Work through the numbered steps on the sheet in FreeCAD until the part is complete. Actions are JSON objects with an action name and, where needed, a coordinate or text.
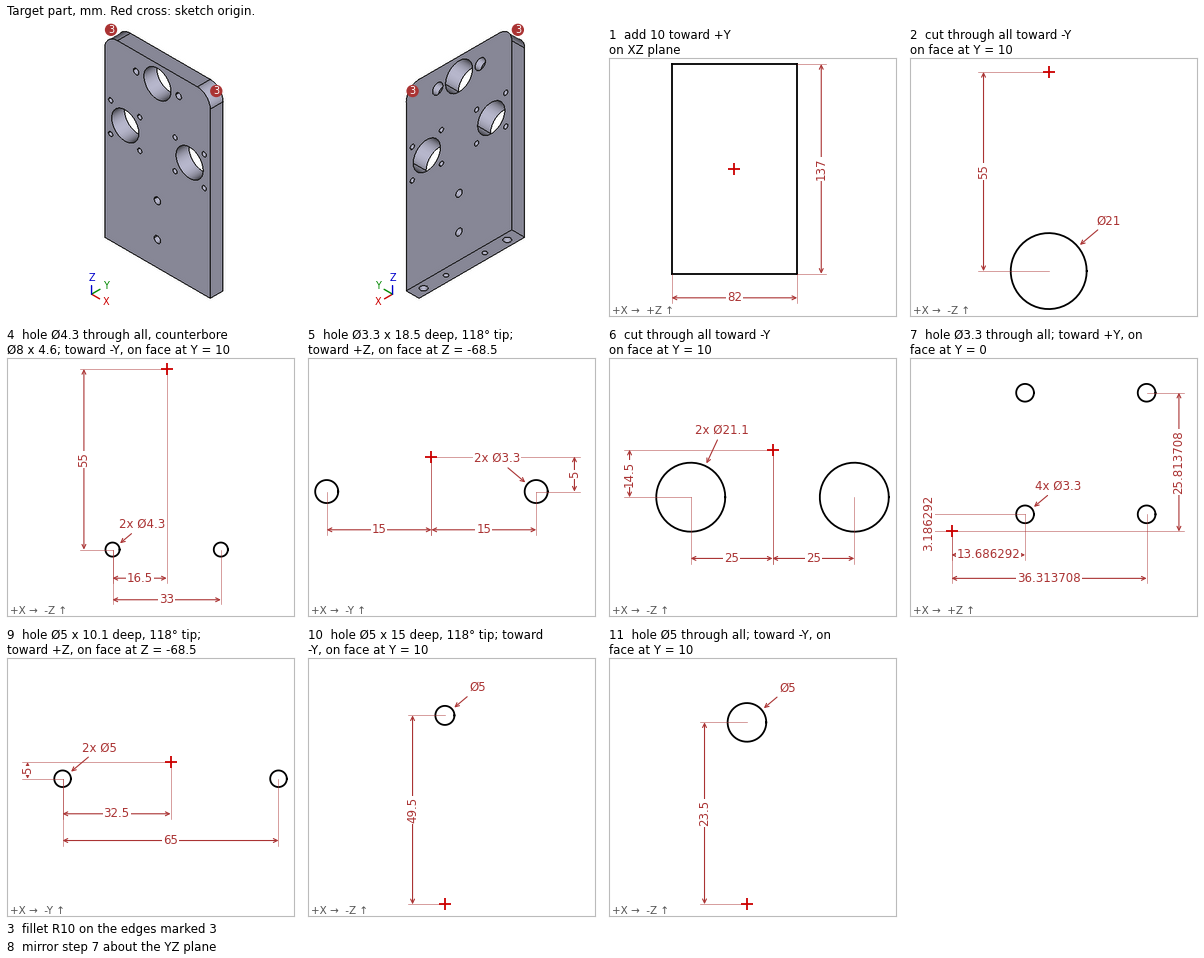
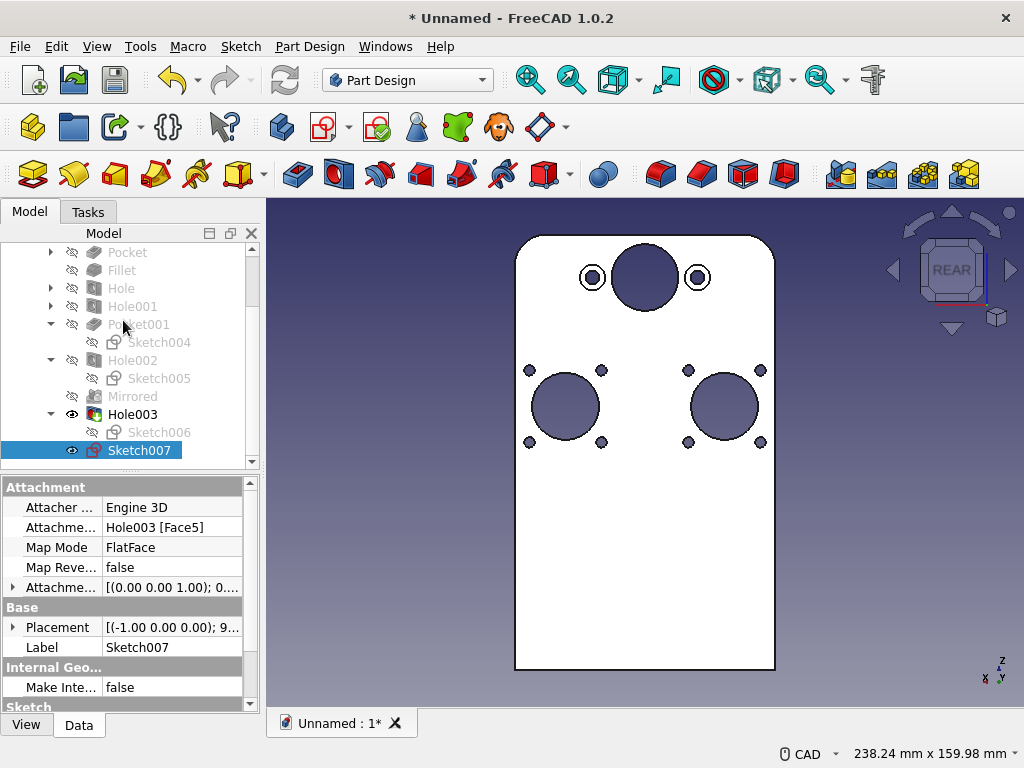
{"action": "left_click", "coordinate": [339, 174]}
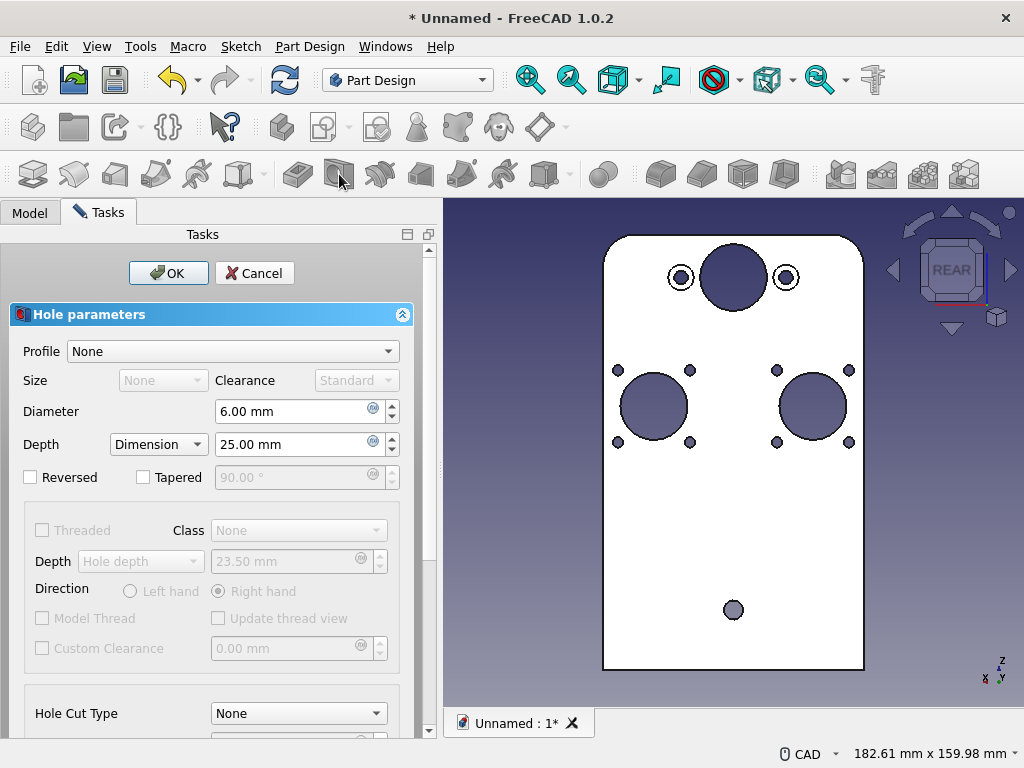
{"action": "triple_click", "coordinate": [300, 412]}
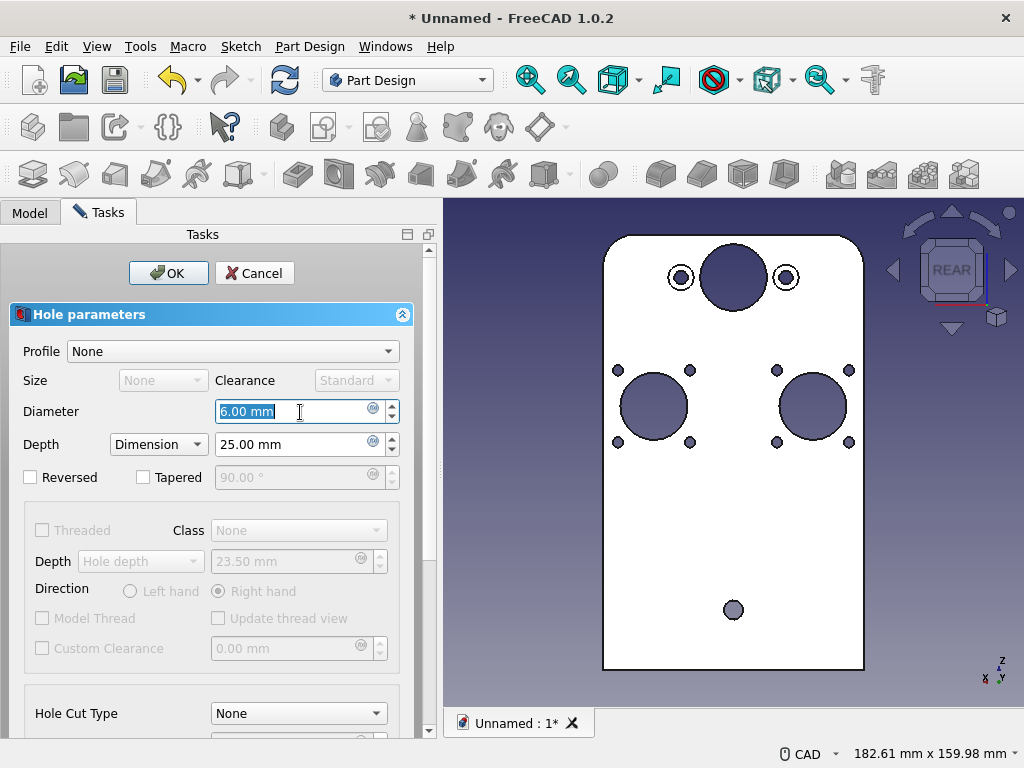
{"action": "type", "text": "5"}
{"action": "key", "text": "Tab"}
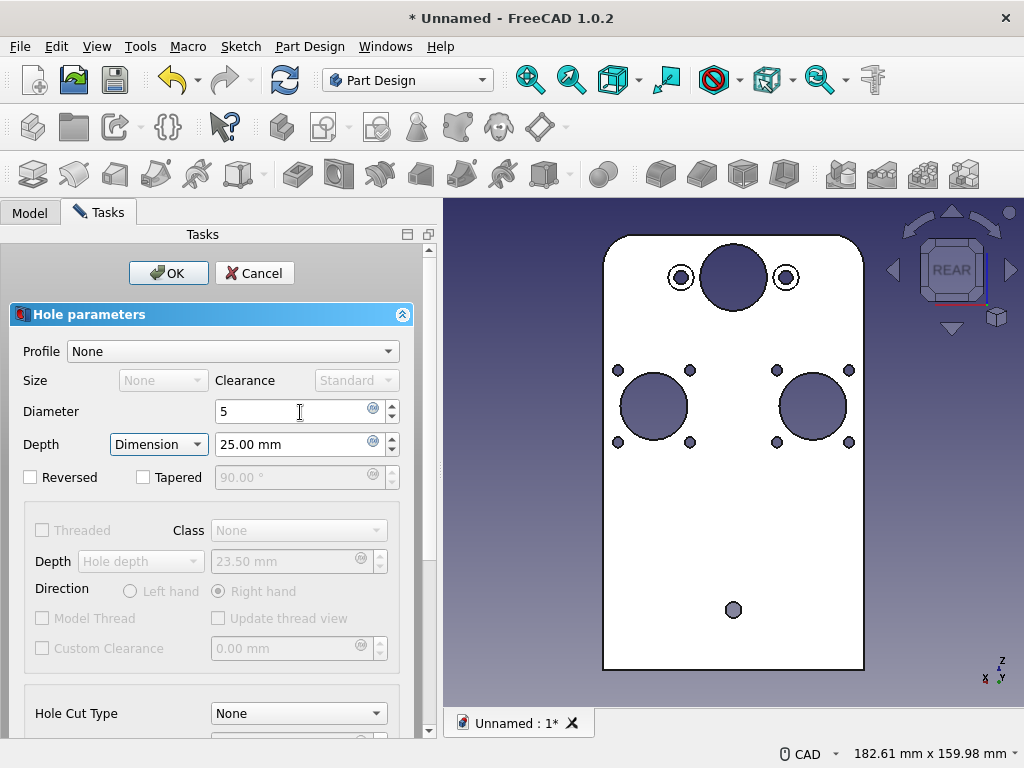
{"action": "triple_click", "coordinate": [300, 444]}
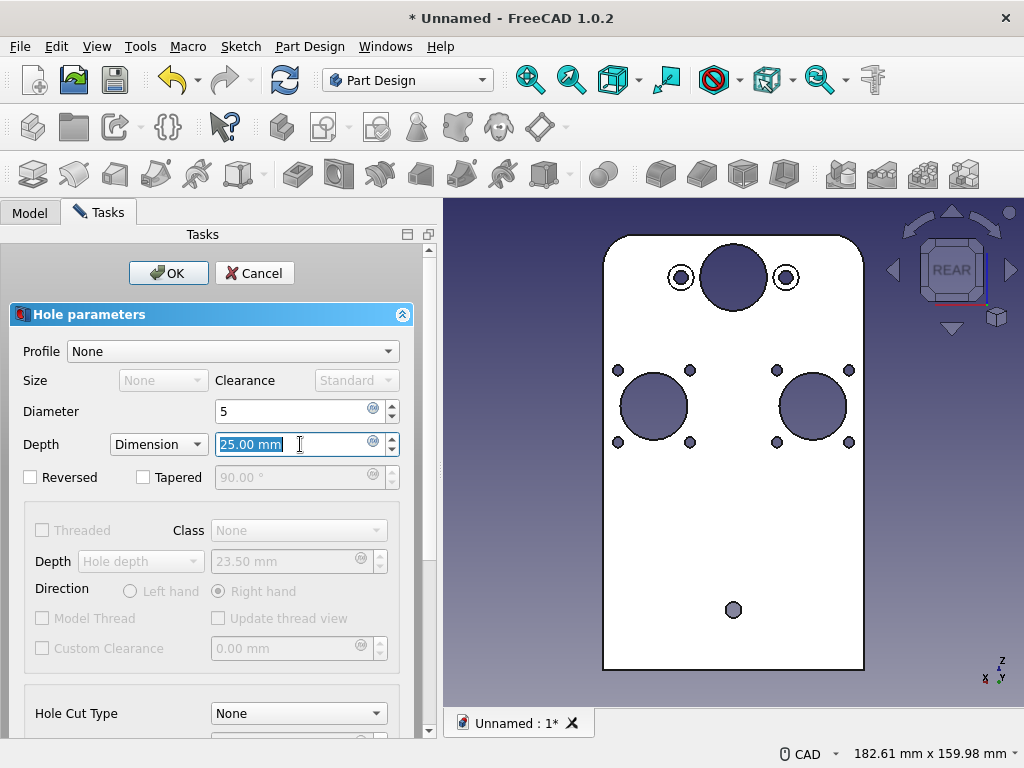
{"action": "type", "text": "15"}
{"action": "key", "text": "Tab"}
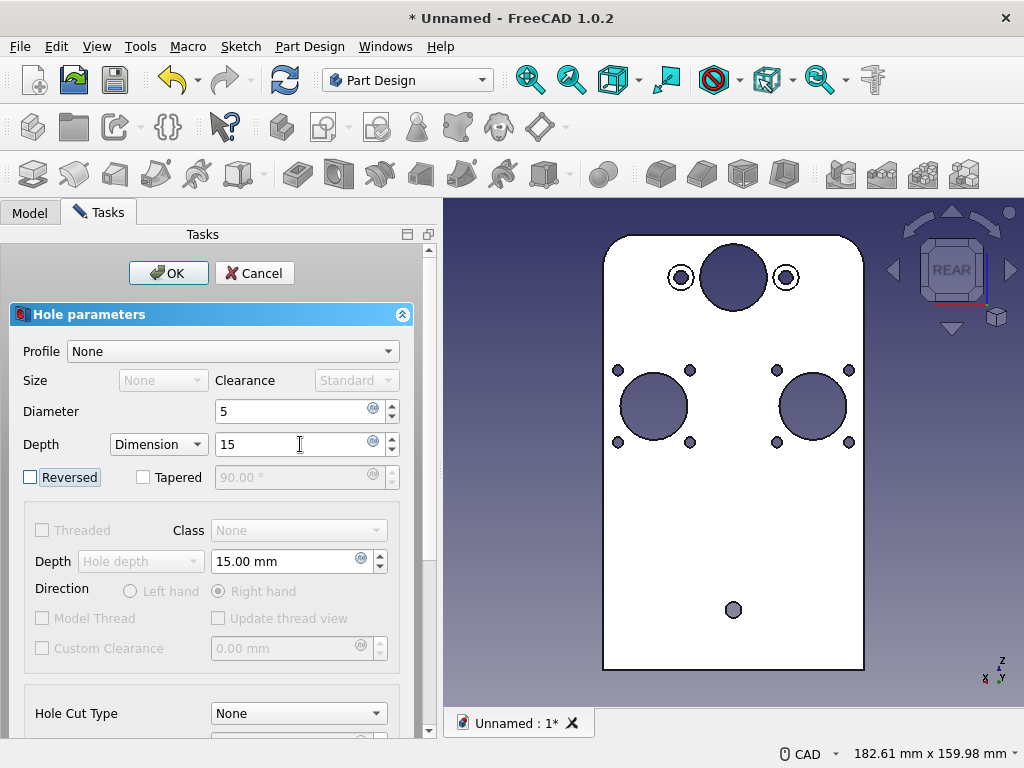
{"action": "left_click", "coordinate": [169, 273]}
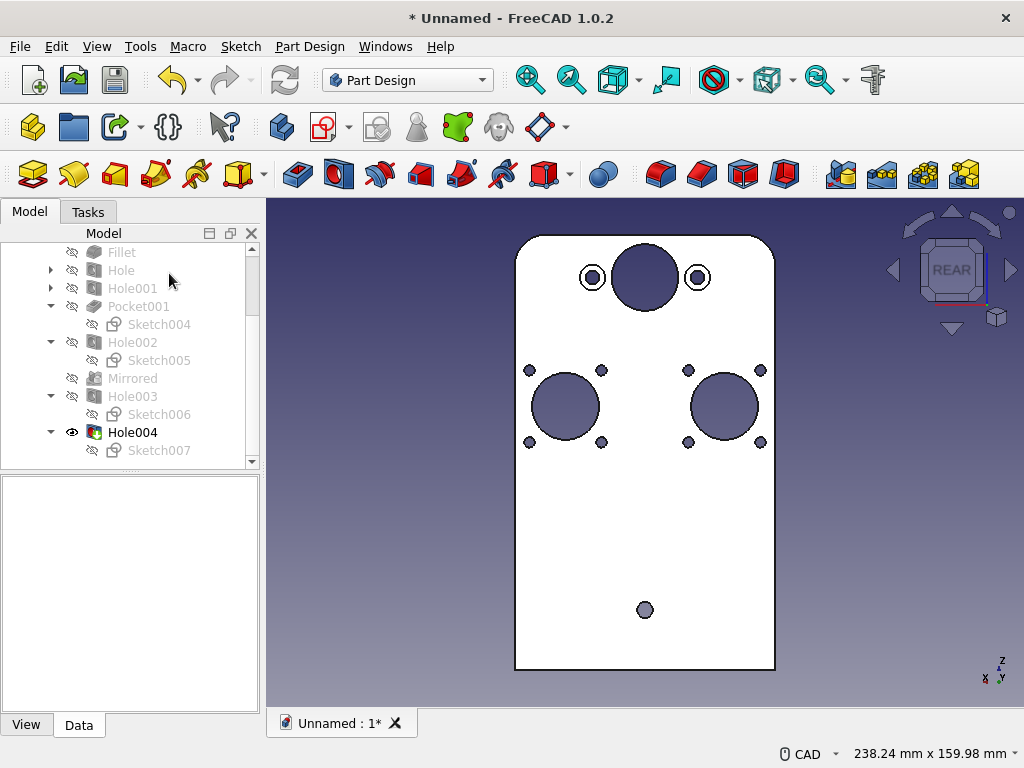
{"action": "left_click", "coordinate": [645, 514]}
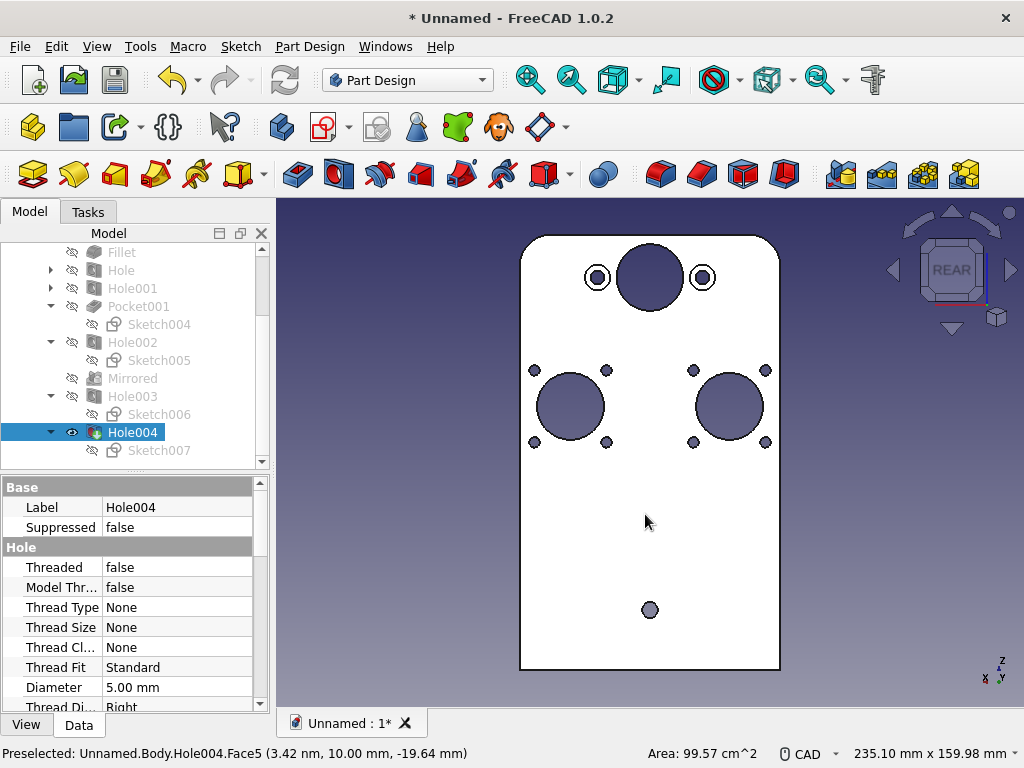
{"action": "left_click", "coordinate": [322, 128]}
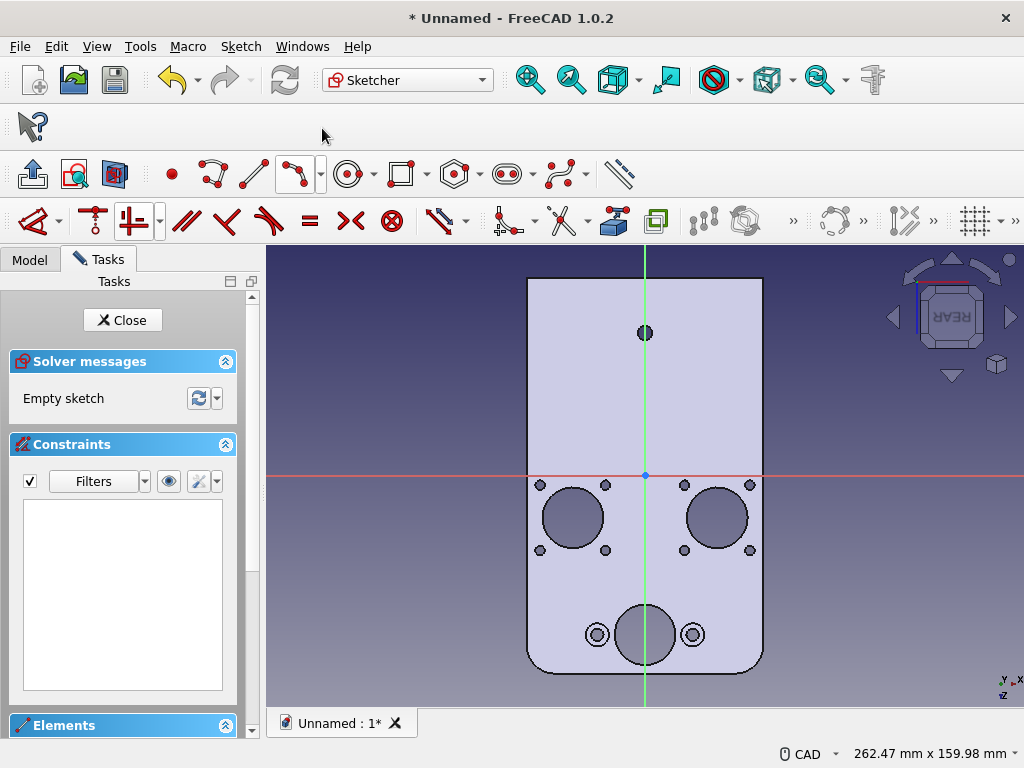
{"action": "scroll", "coordinate": [649, 405], "scroll_direction": "up", "scroll_amount": 15}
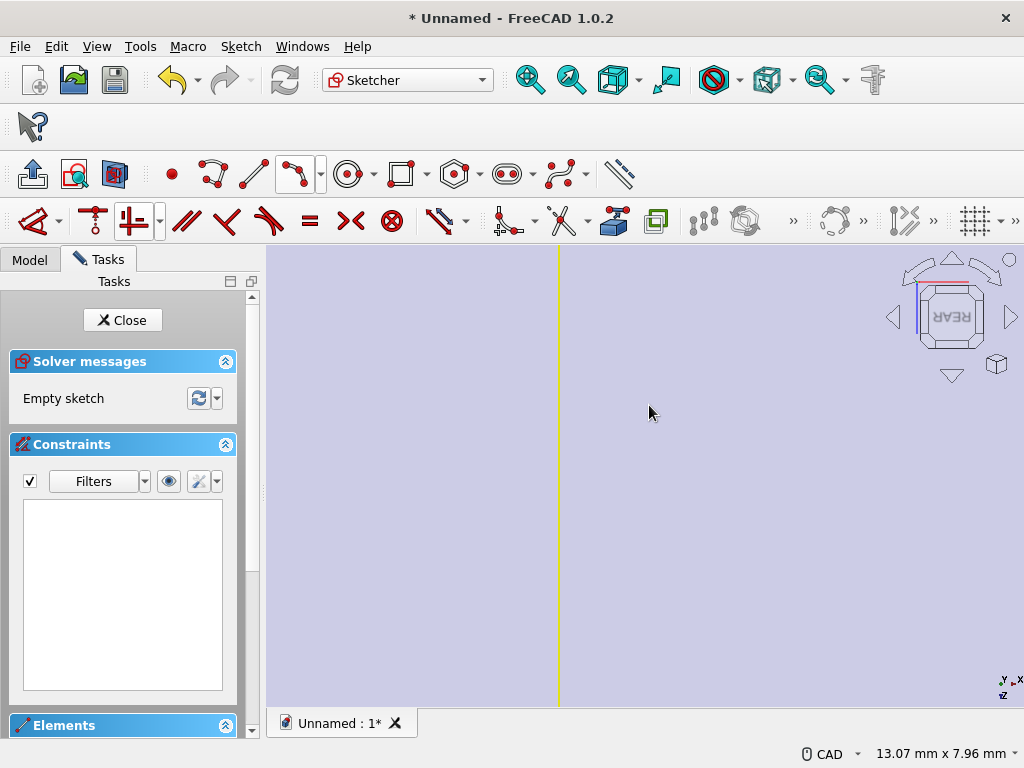
{"action": "key", "text": "g c"}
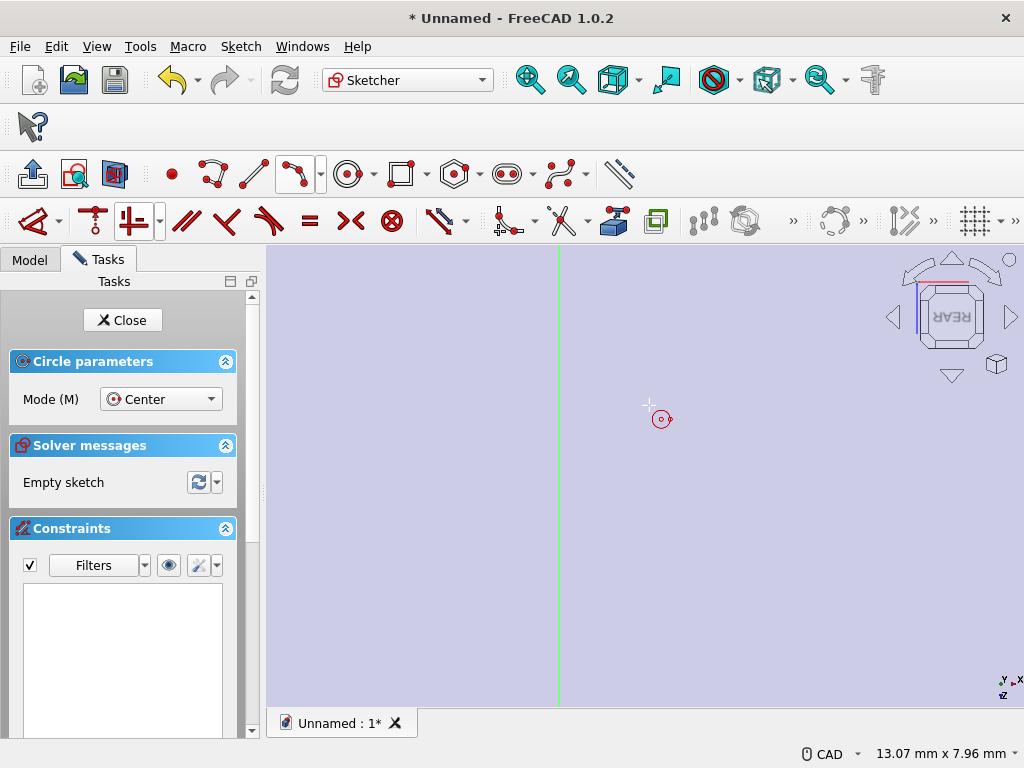
{"action": "left_click", "coordinate": [559, 461]}
{"action": "mouse_move", "coordinate": [662, 359]}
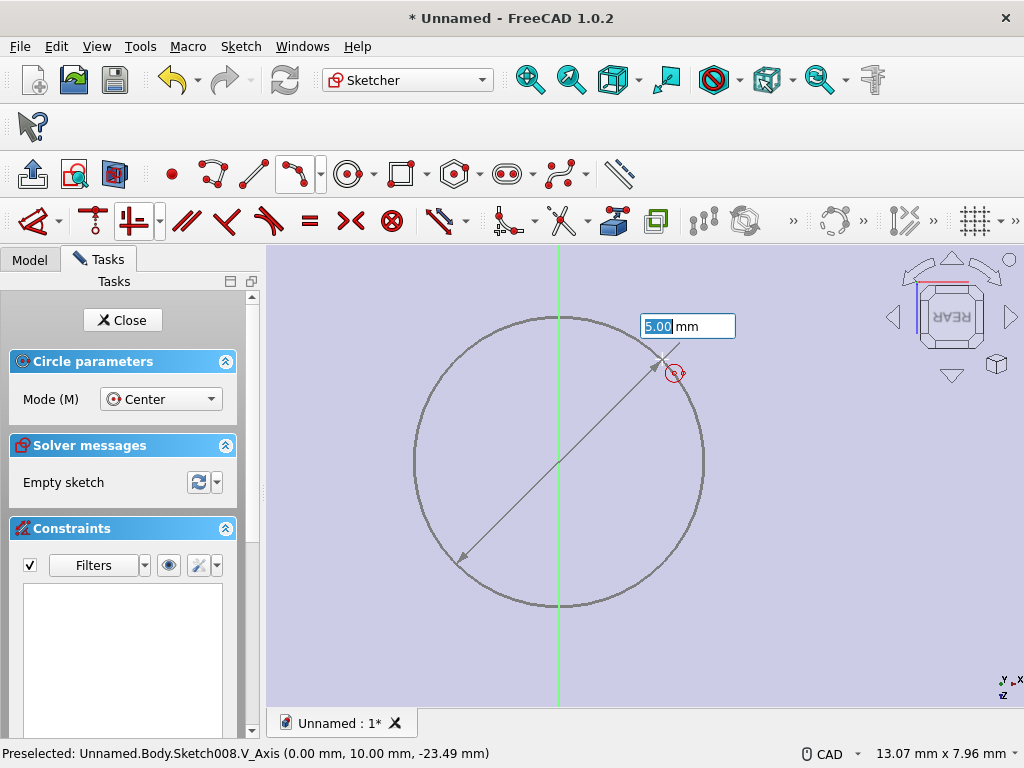
{"action": "type", "text": "5"}
{"action": "key", "text": "Return"}
{"action": "key", "text": "Escape"}